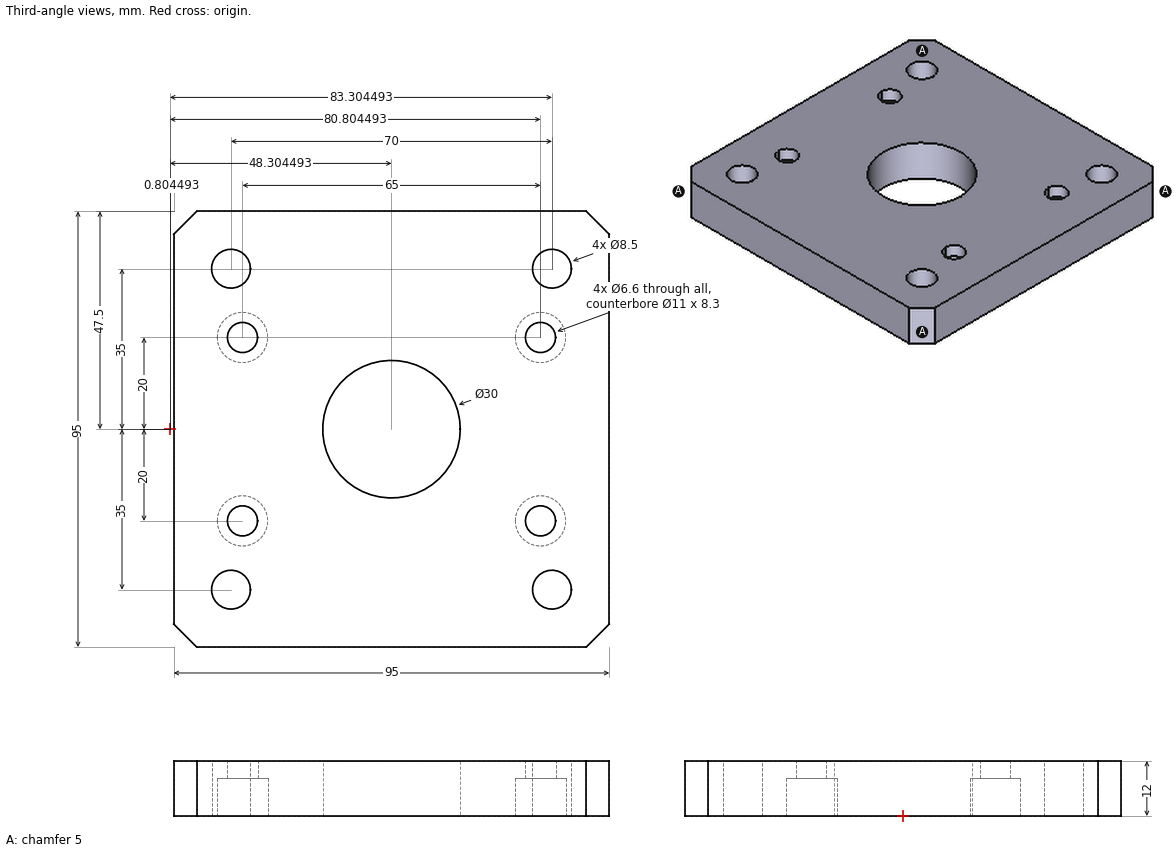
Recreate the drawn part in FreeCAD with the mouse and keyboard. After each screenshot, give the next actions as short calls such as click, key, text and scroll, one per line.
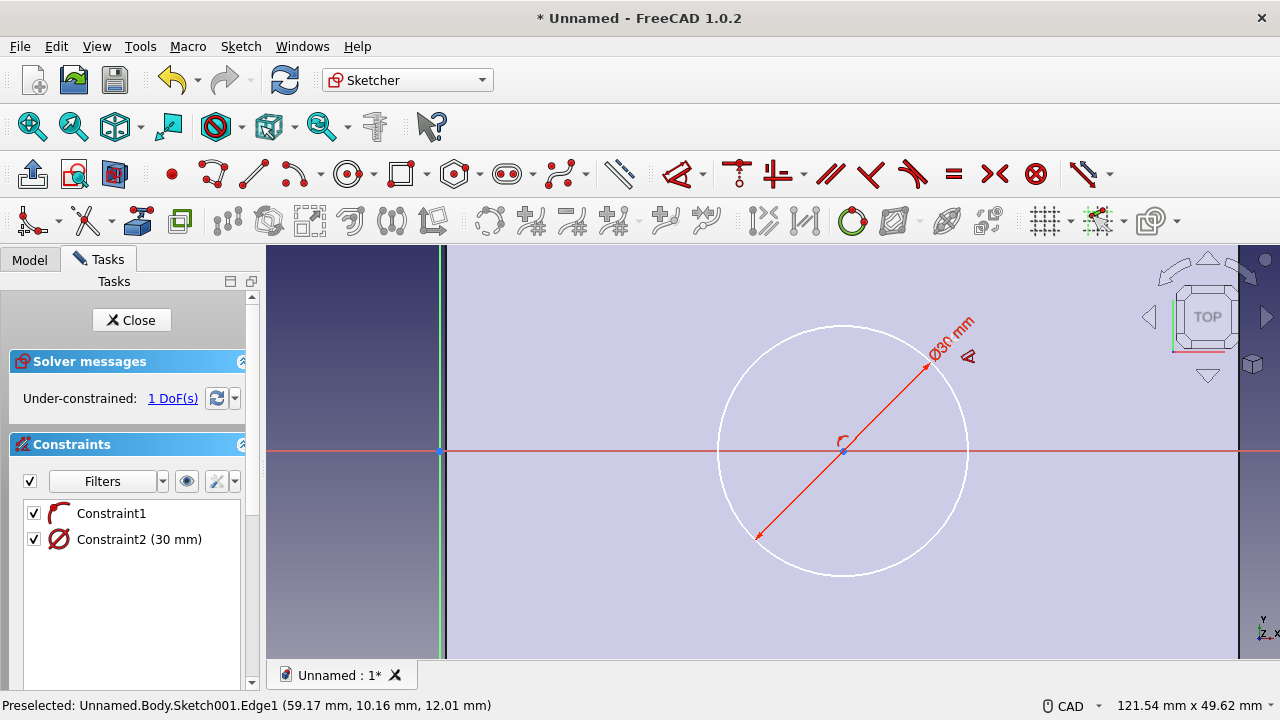
click(843, 451)
click(641, 485)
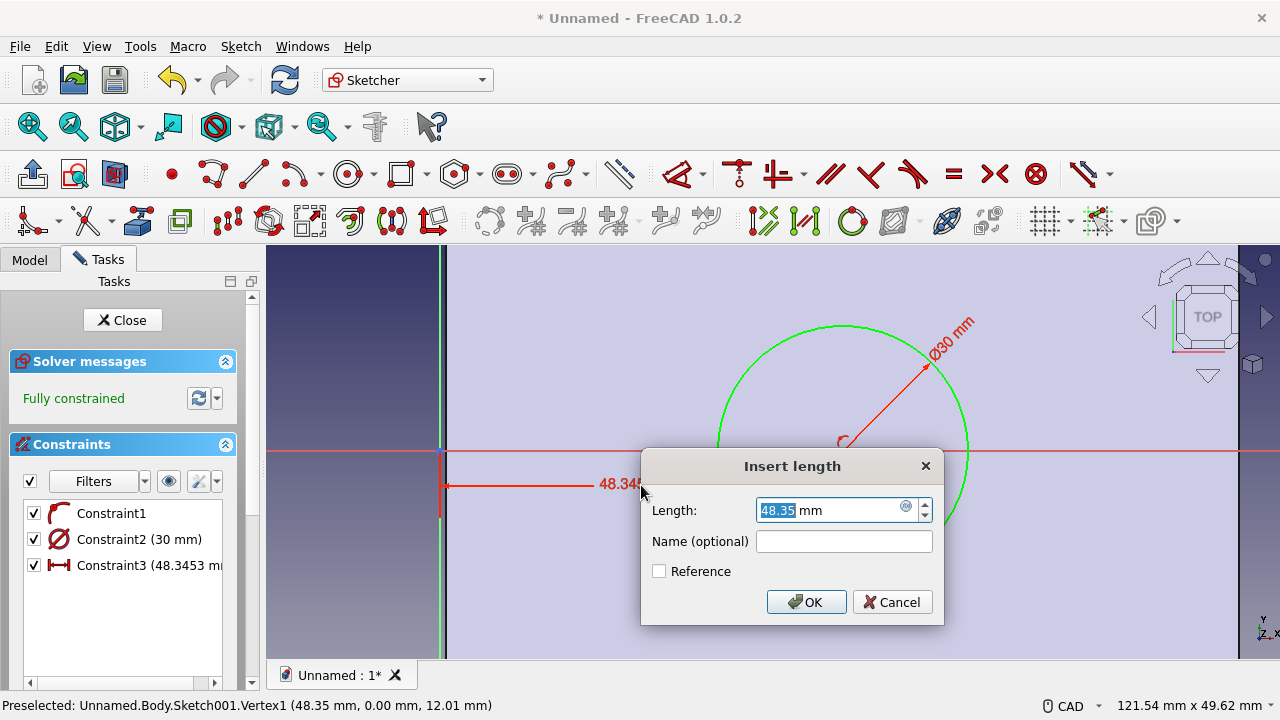
text(48.304493)
key(Return)
key(Escape)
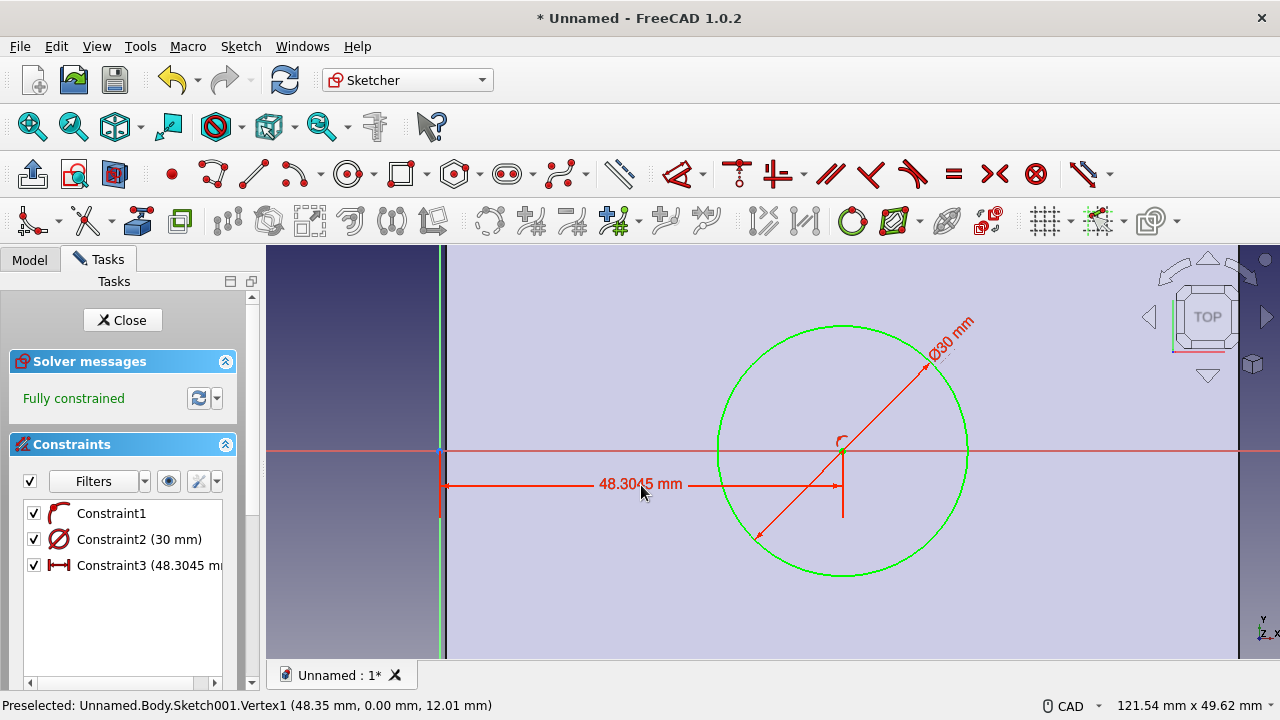
click(123, 320)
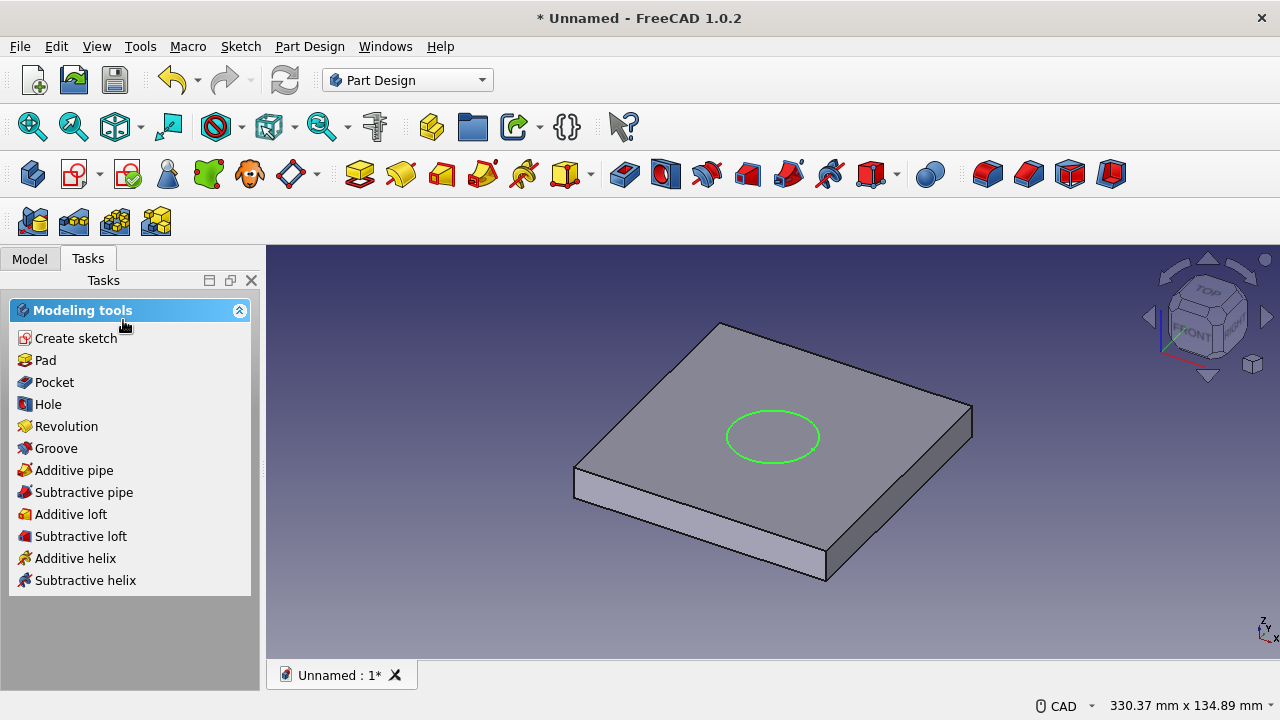
click(625, 174)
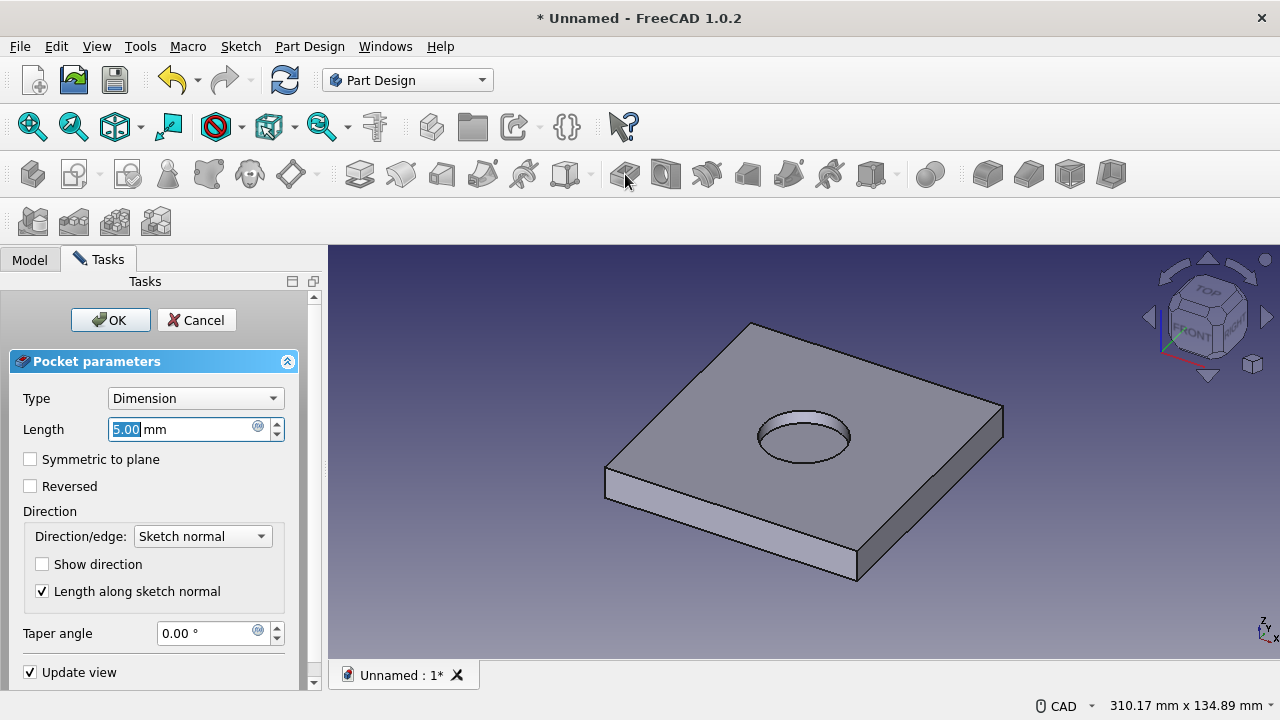
click(196, 398)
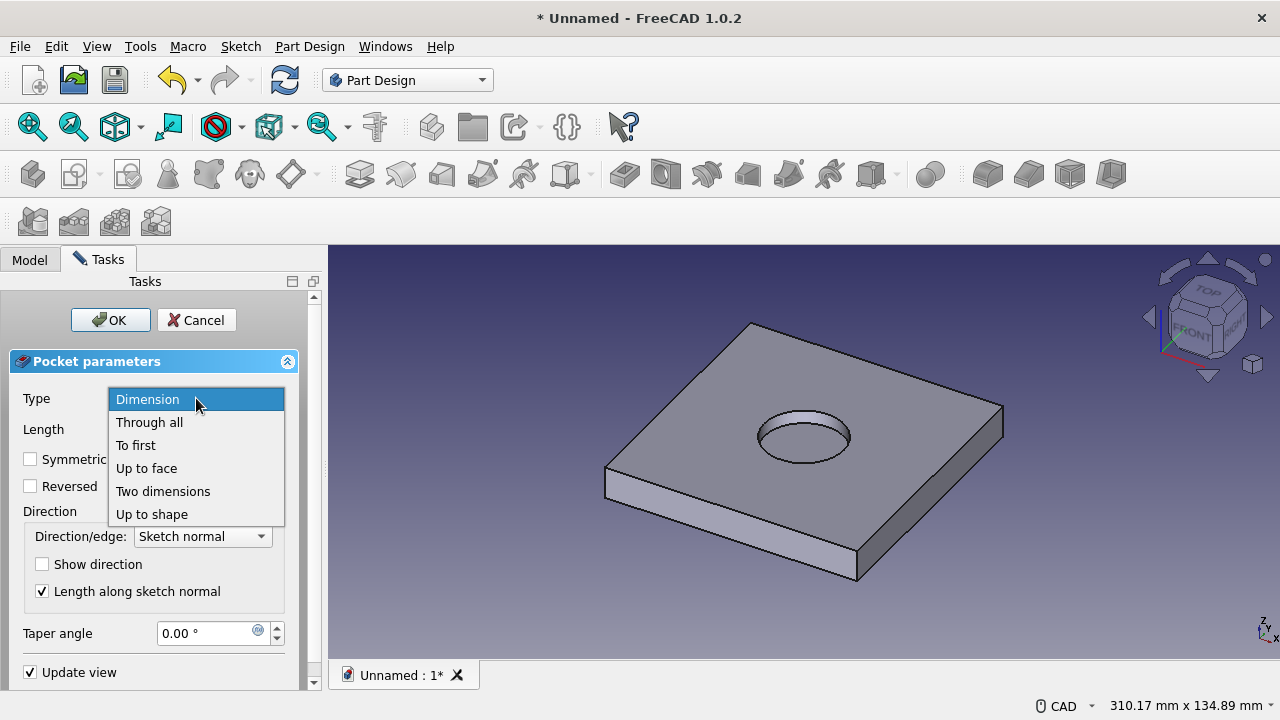
click(194, 422)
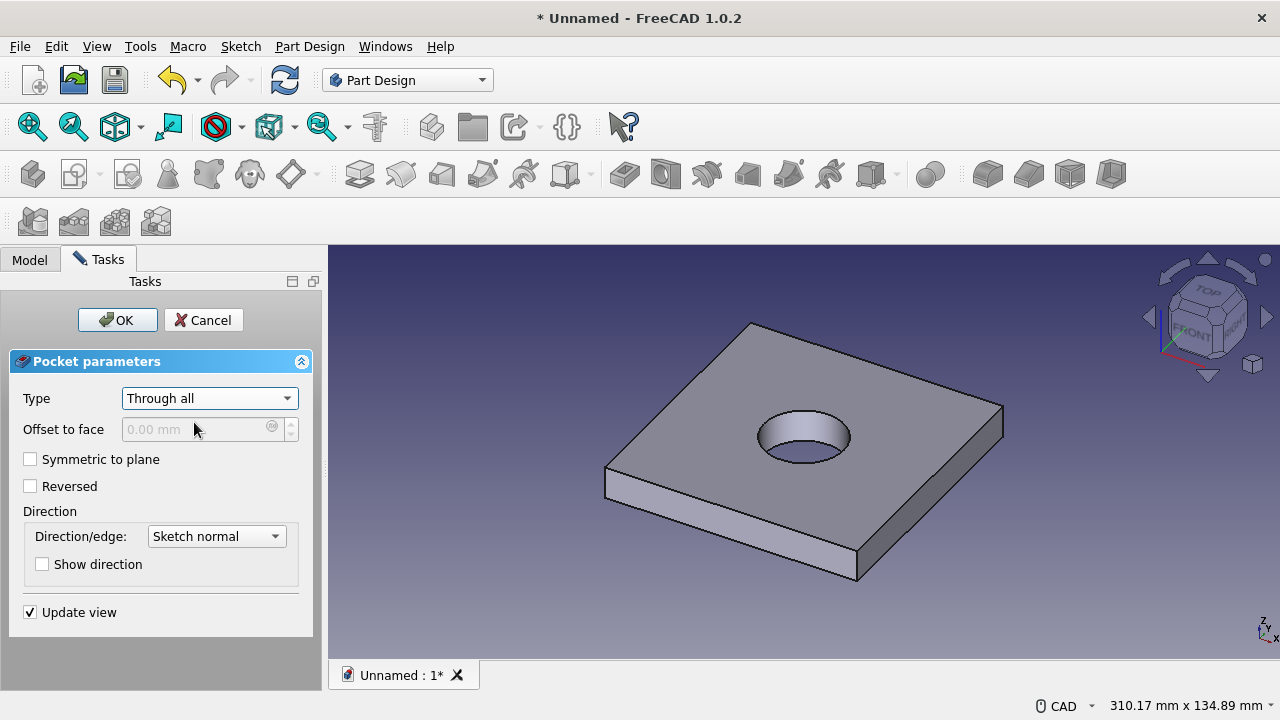
click(118, 320)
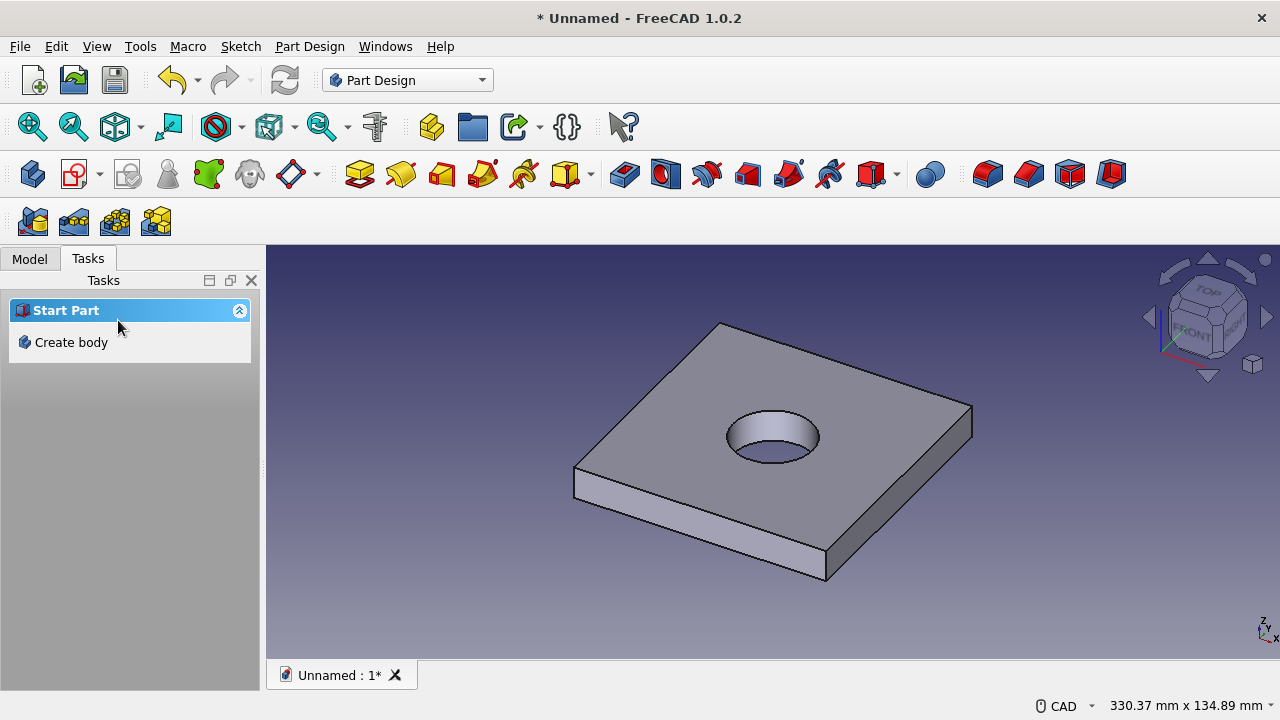
click(74, 174)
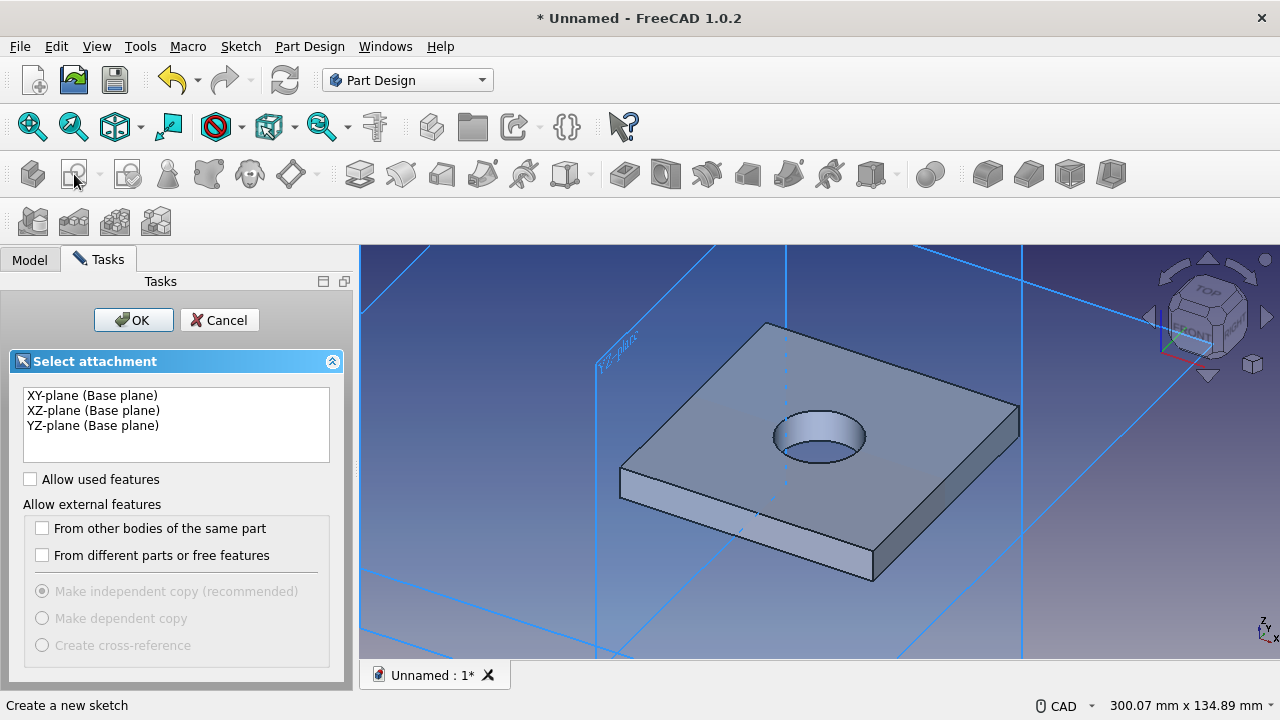
click(84, 396)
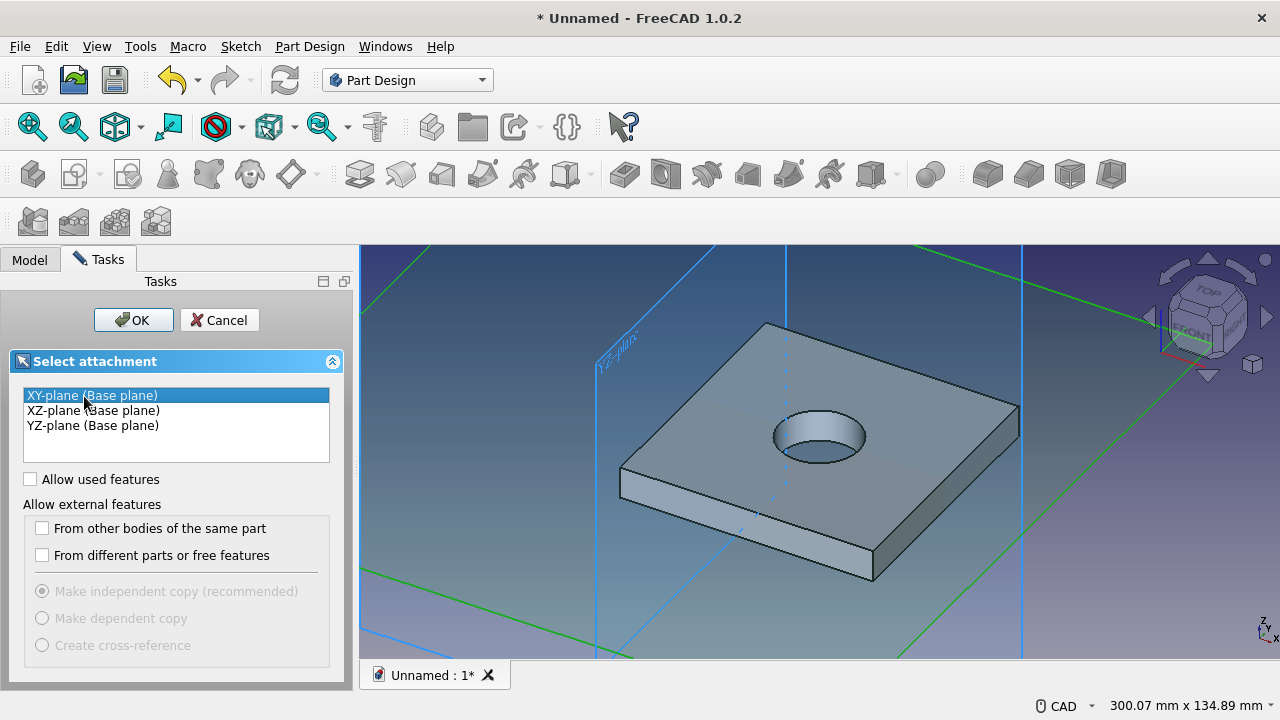
click(134, 320)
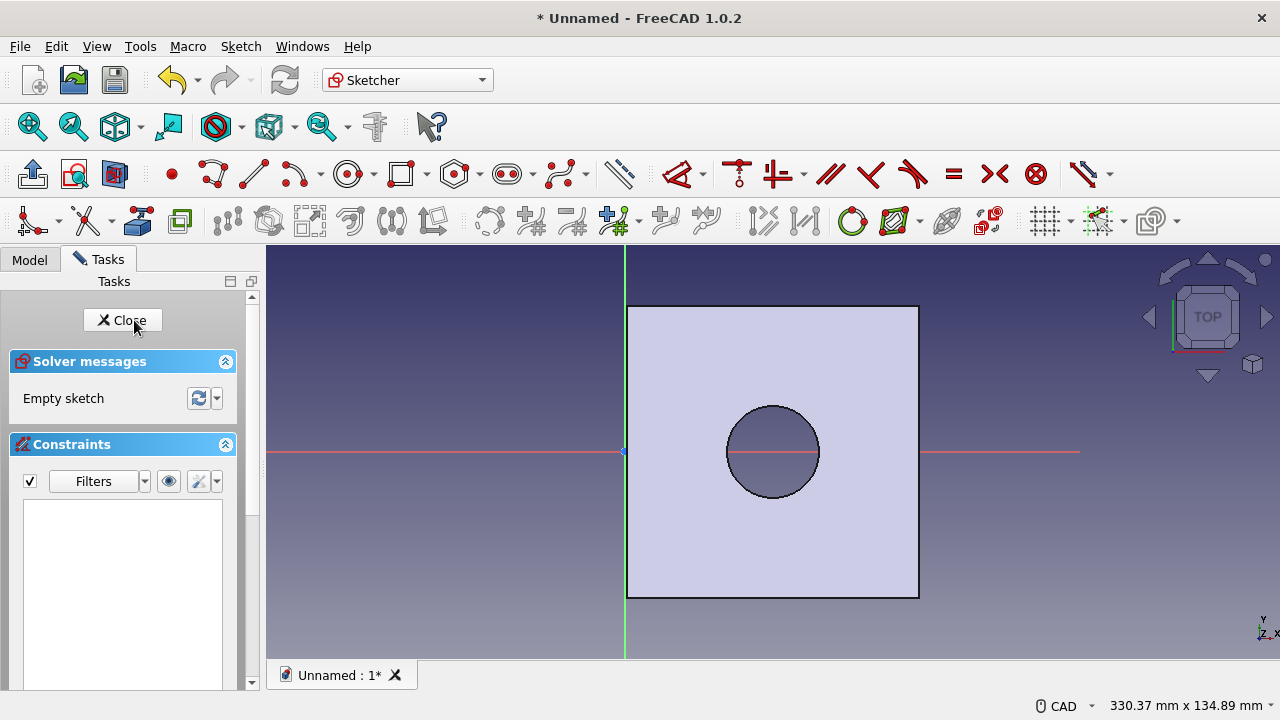
click(115, 174)